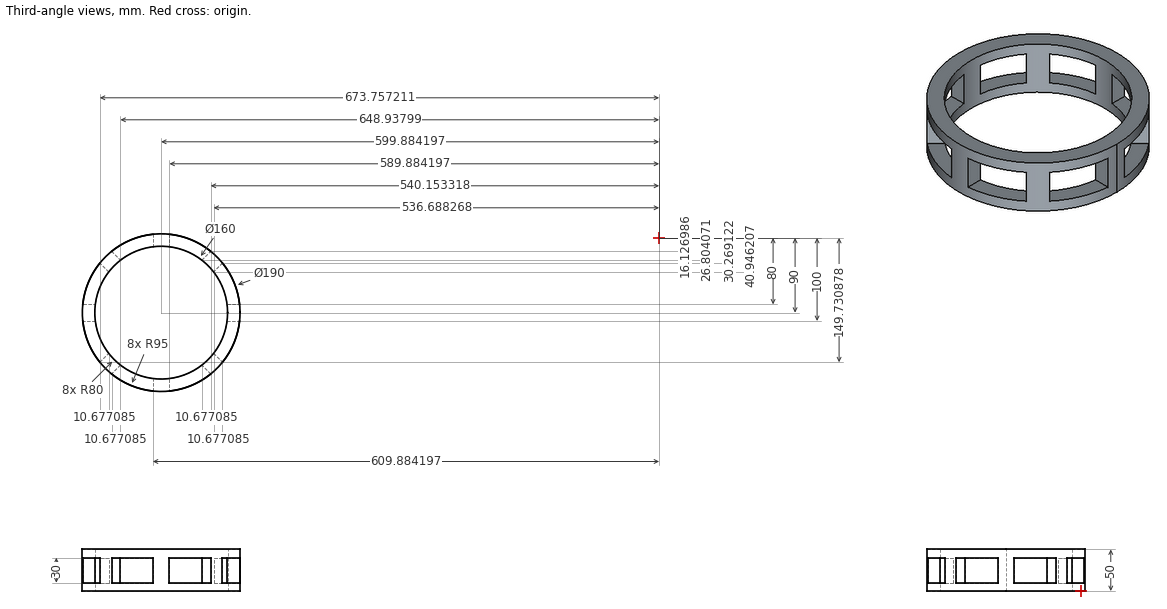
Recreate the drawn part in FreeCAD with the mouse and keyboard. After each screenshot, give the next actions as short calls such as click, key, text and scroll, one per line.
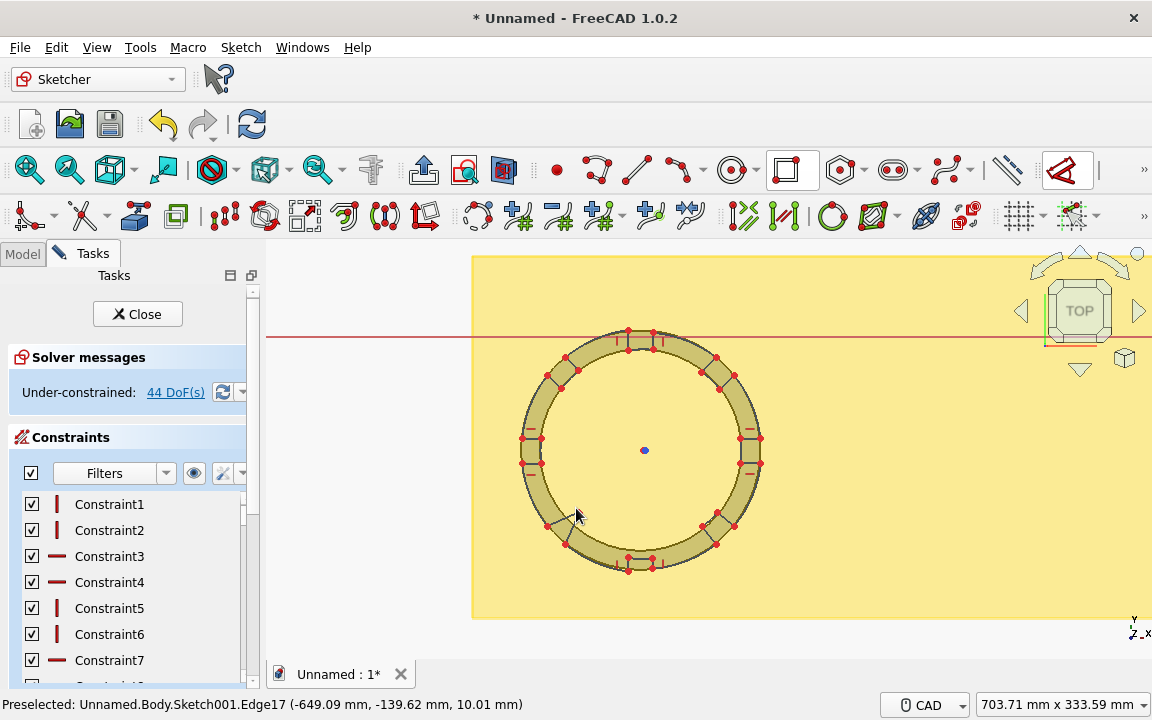
click(526, 484)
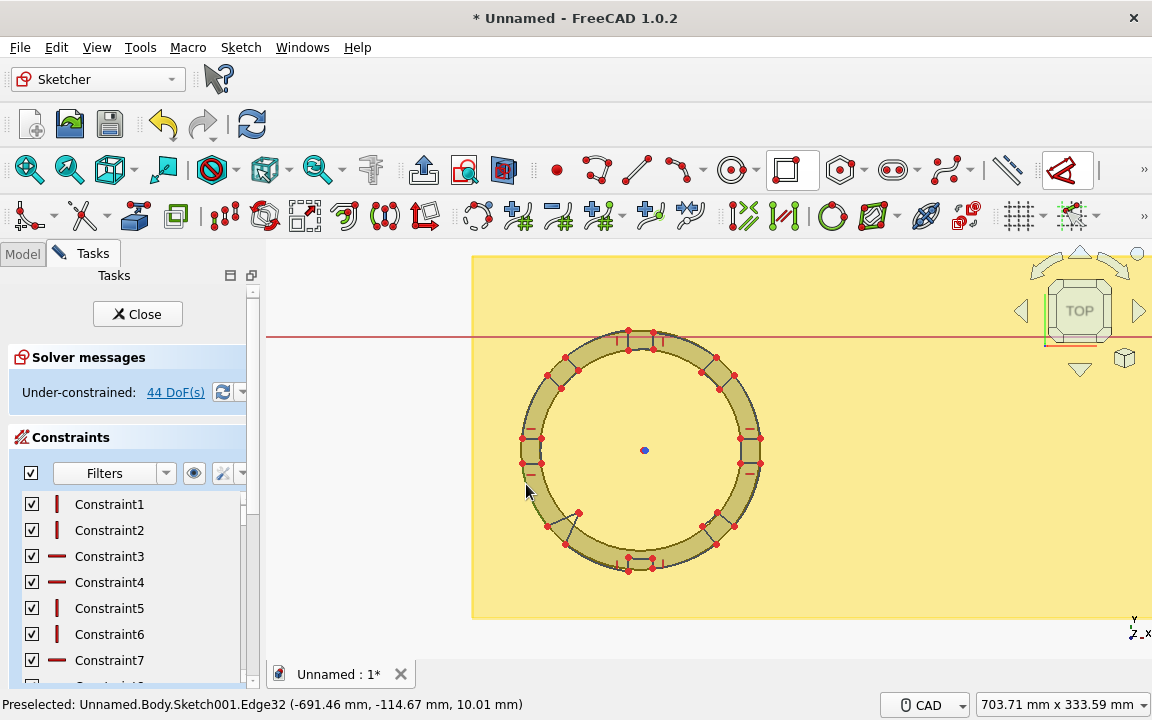
key(c)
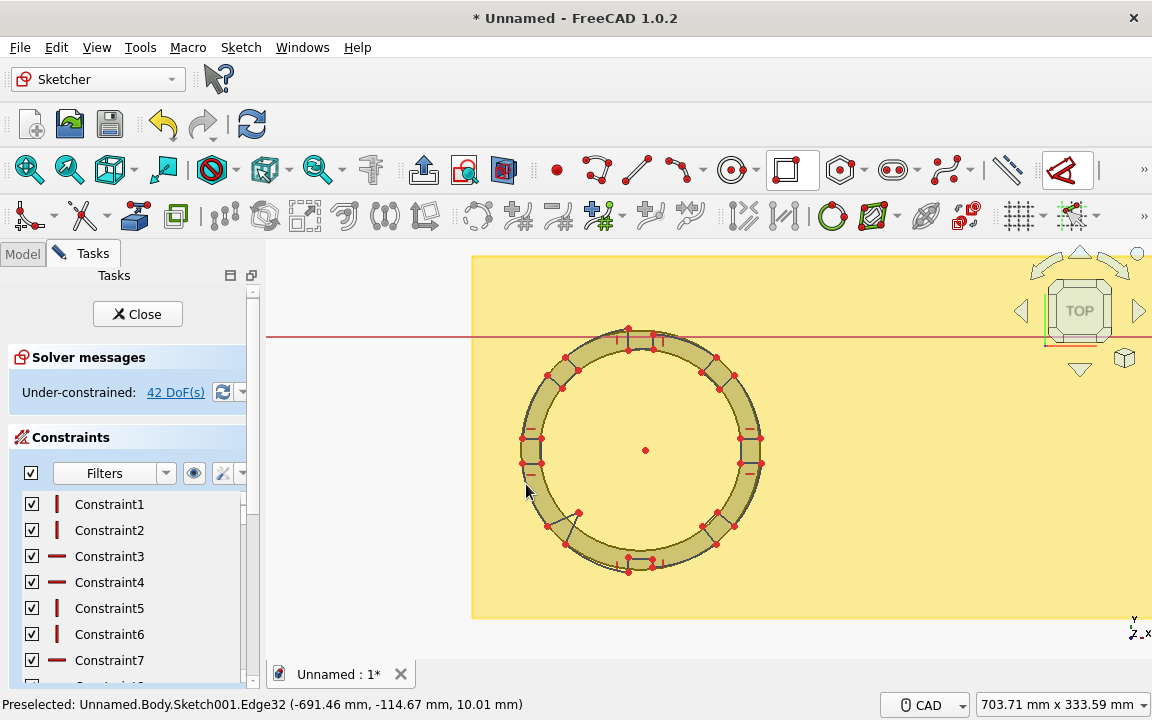
scroll(579, 513, up, 15)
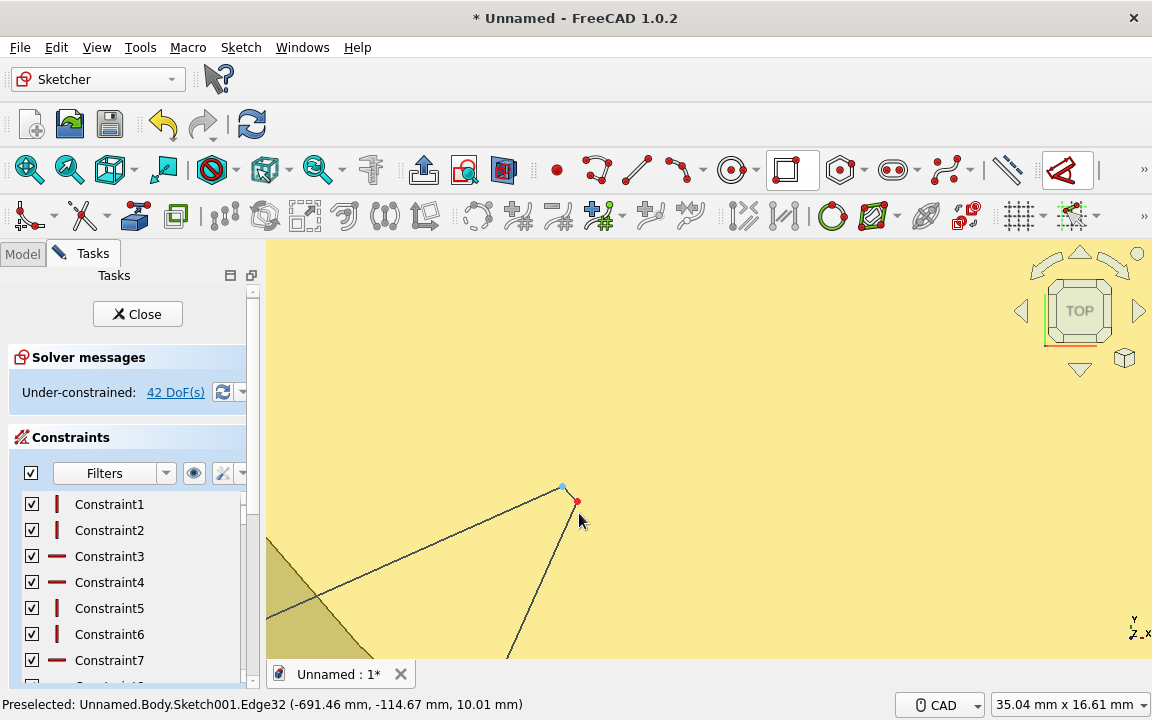
click(570, 494)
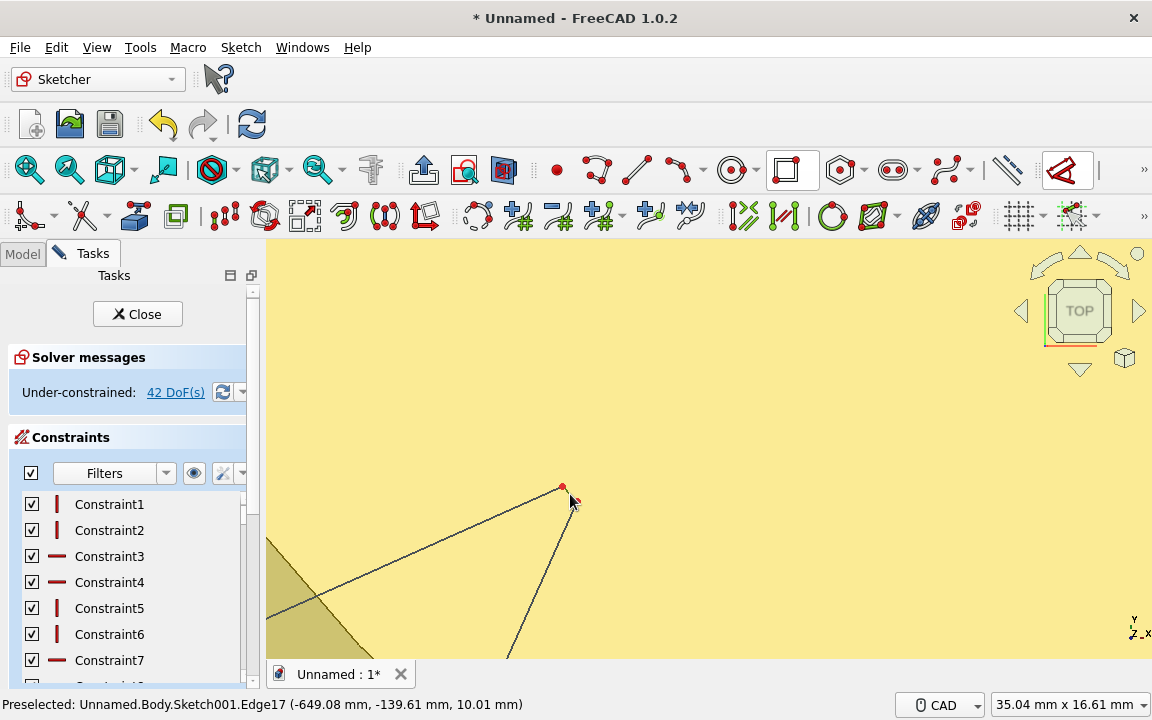
scroll(579, 513, down, 15)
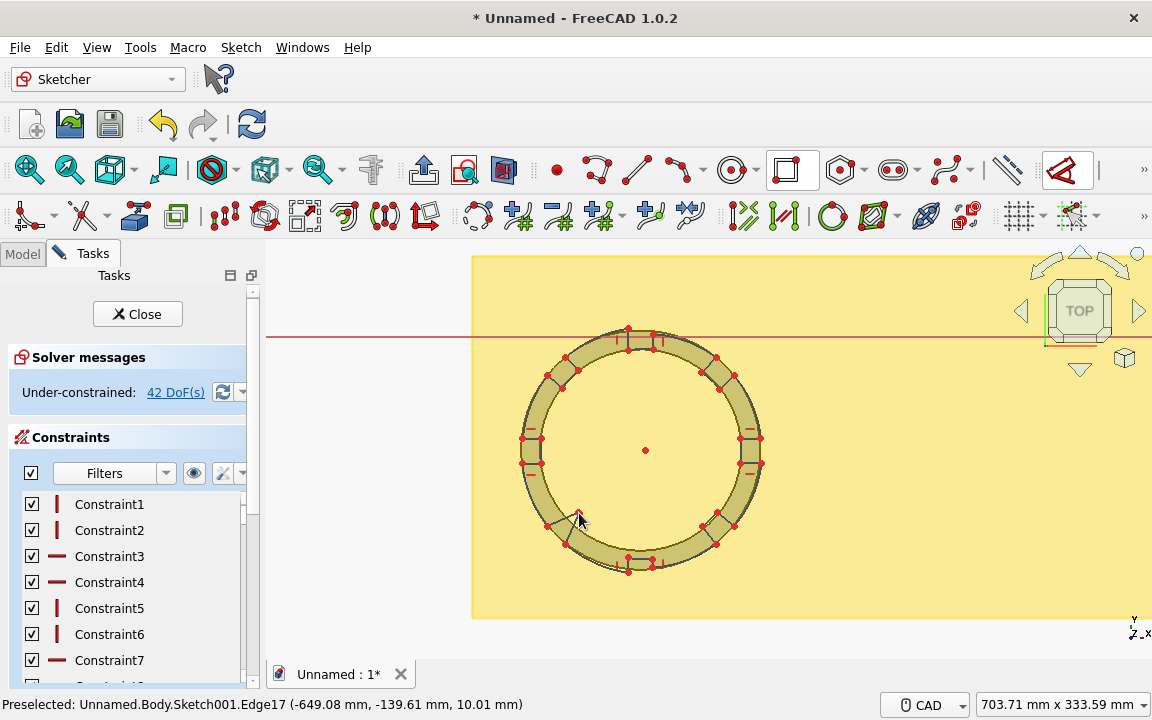
scroll(636, 559, up, 4)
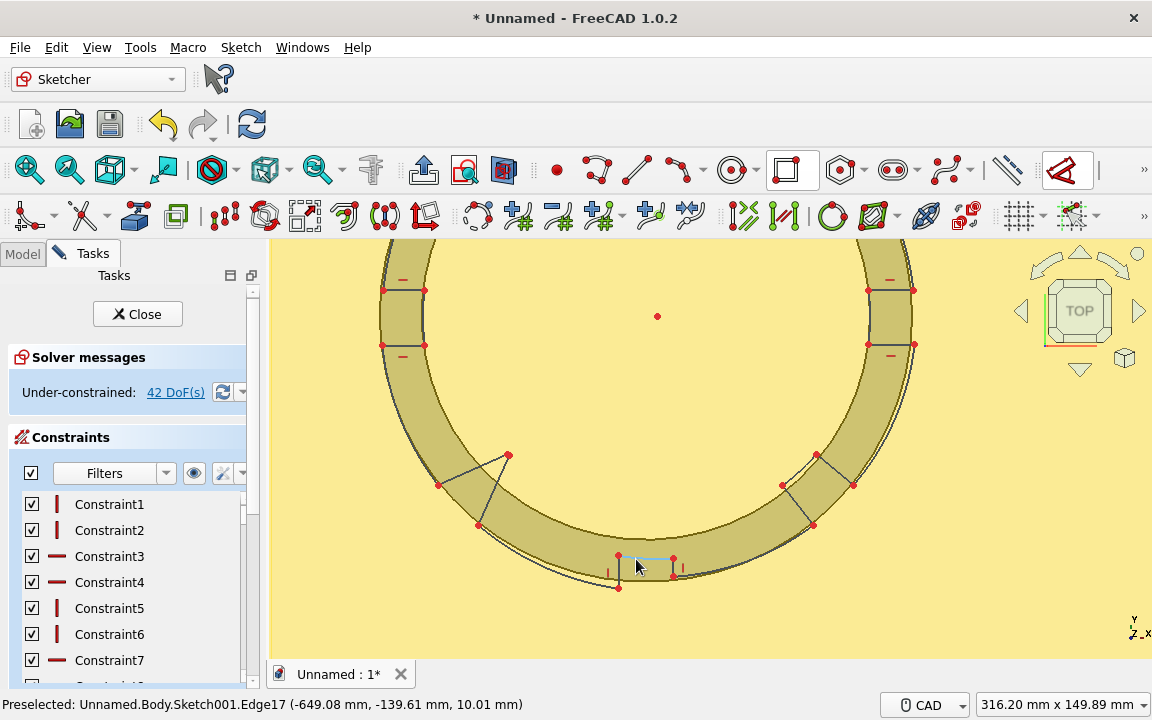
click(635, 558)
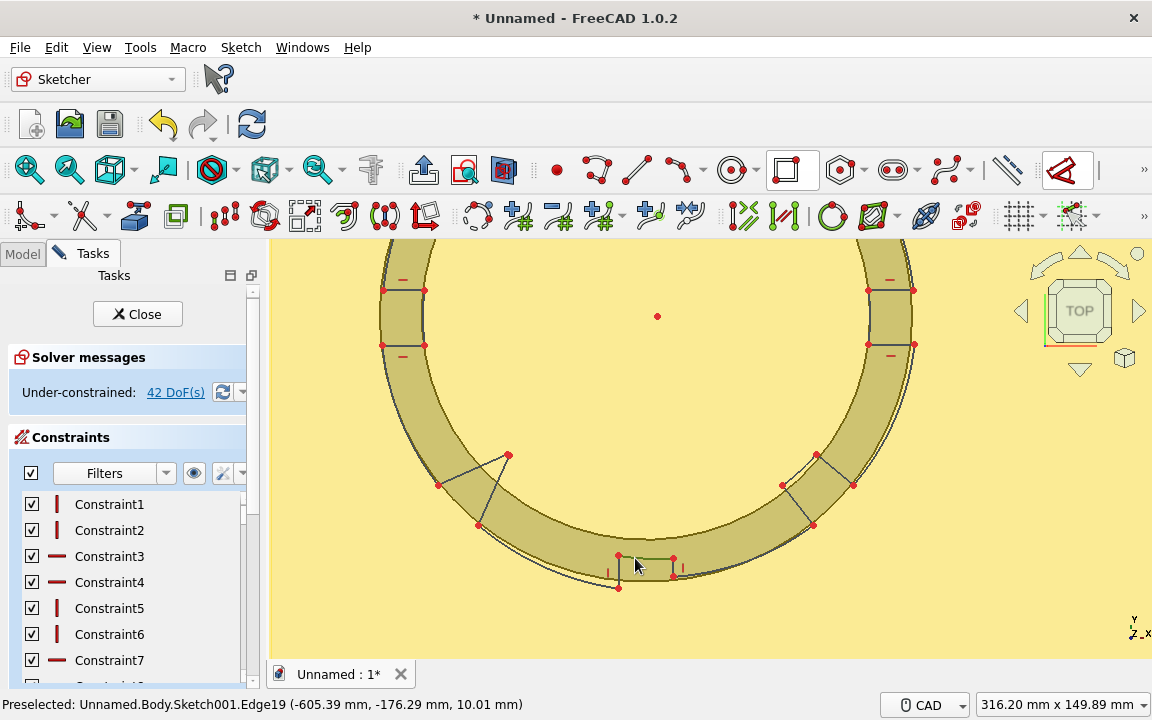
click(793, 477)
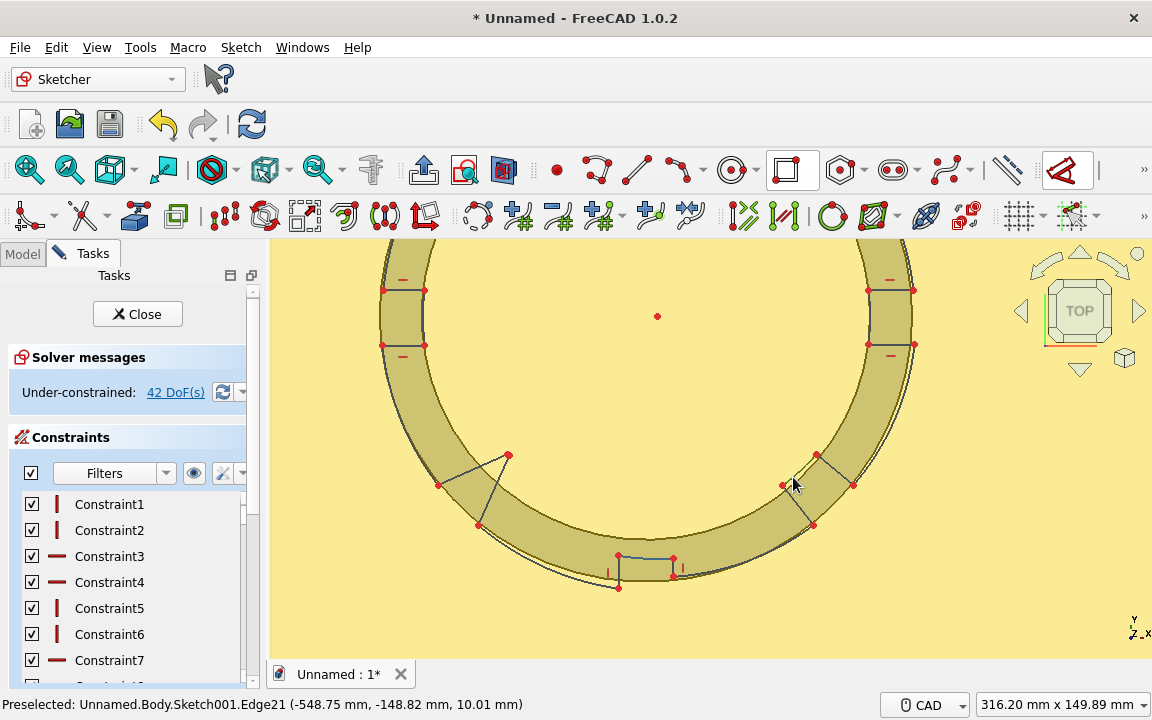
click(870, 328)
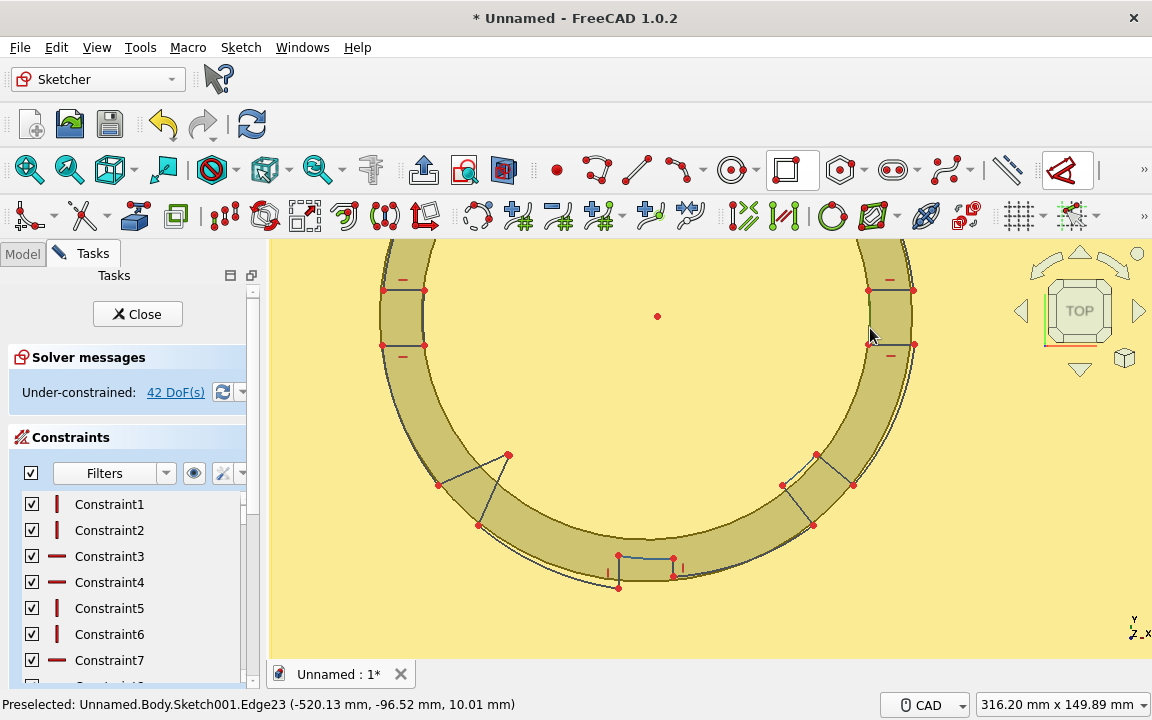
scroll(636, 558, down, 4)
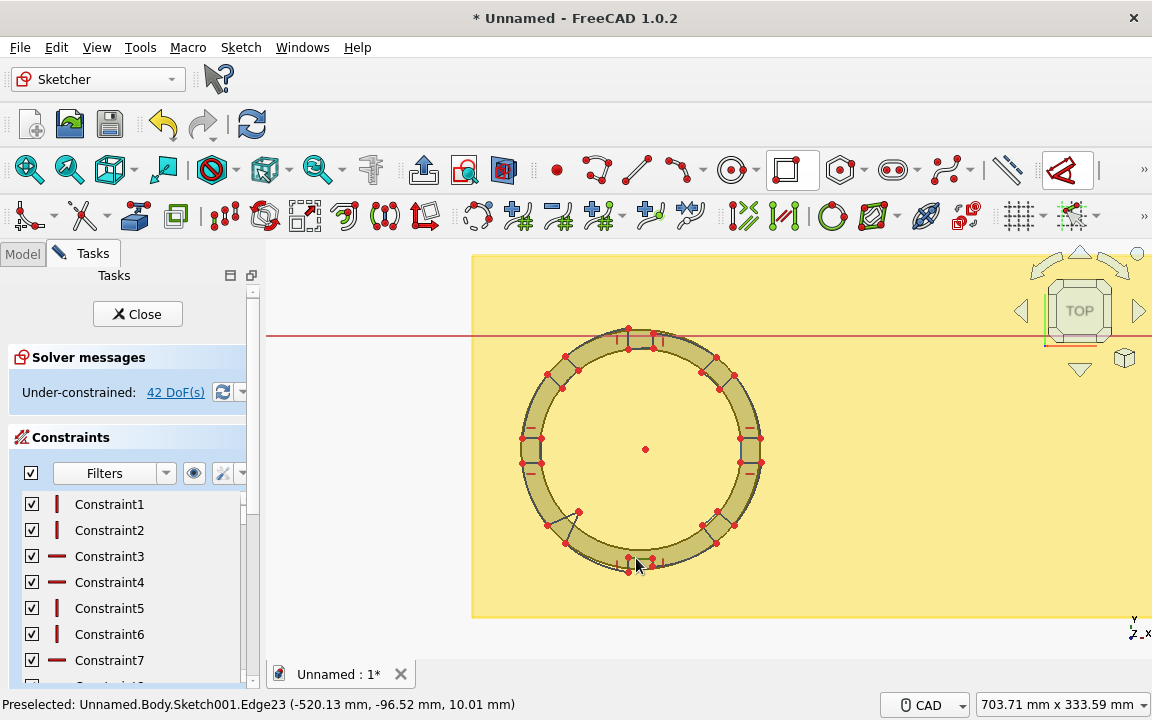
scroll(715, 383, up, 4)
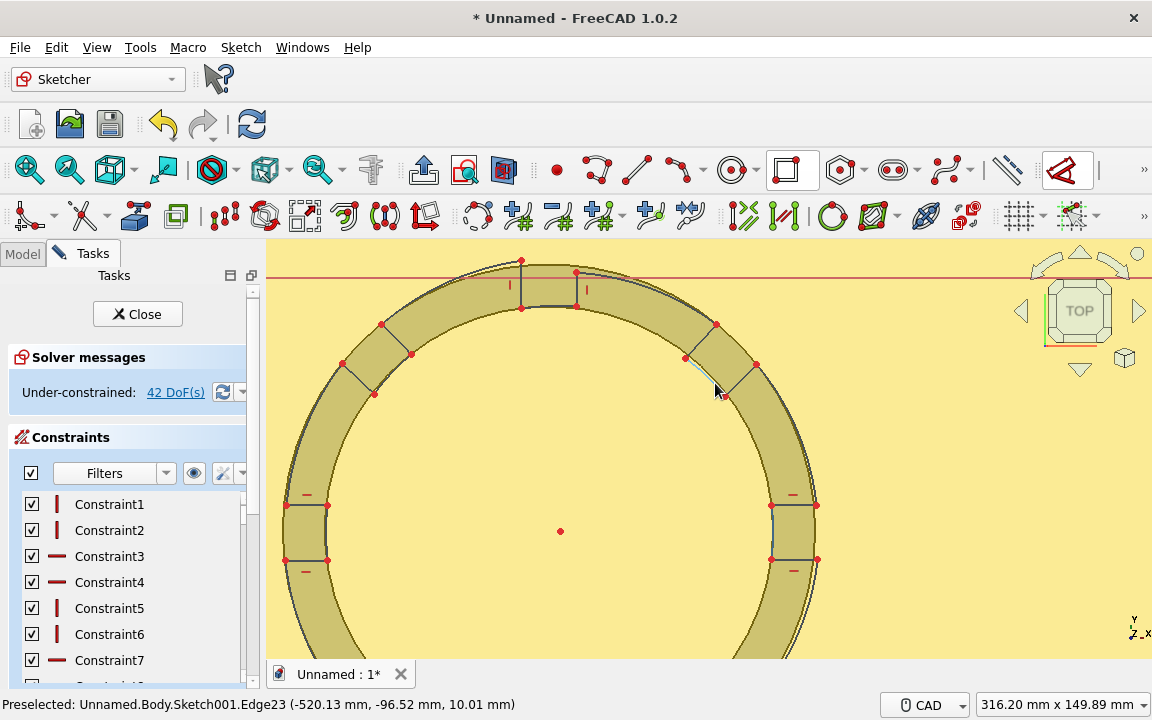
click(714, 384)